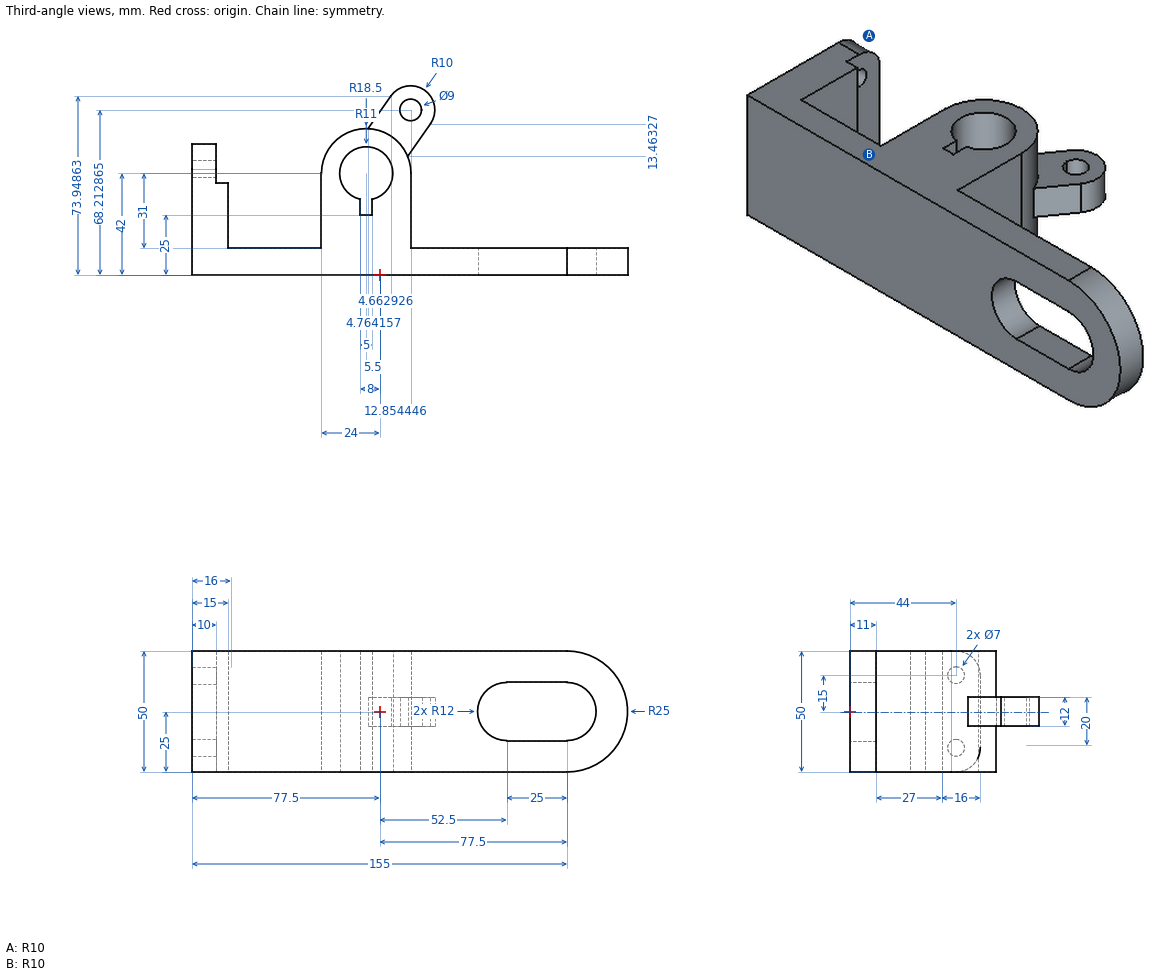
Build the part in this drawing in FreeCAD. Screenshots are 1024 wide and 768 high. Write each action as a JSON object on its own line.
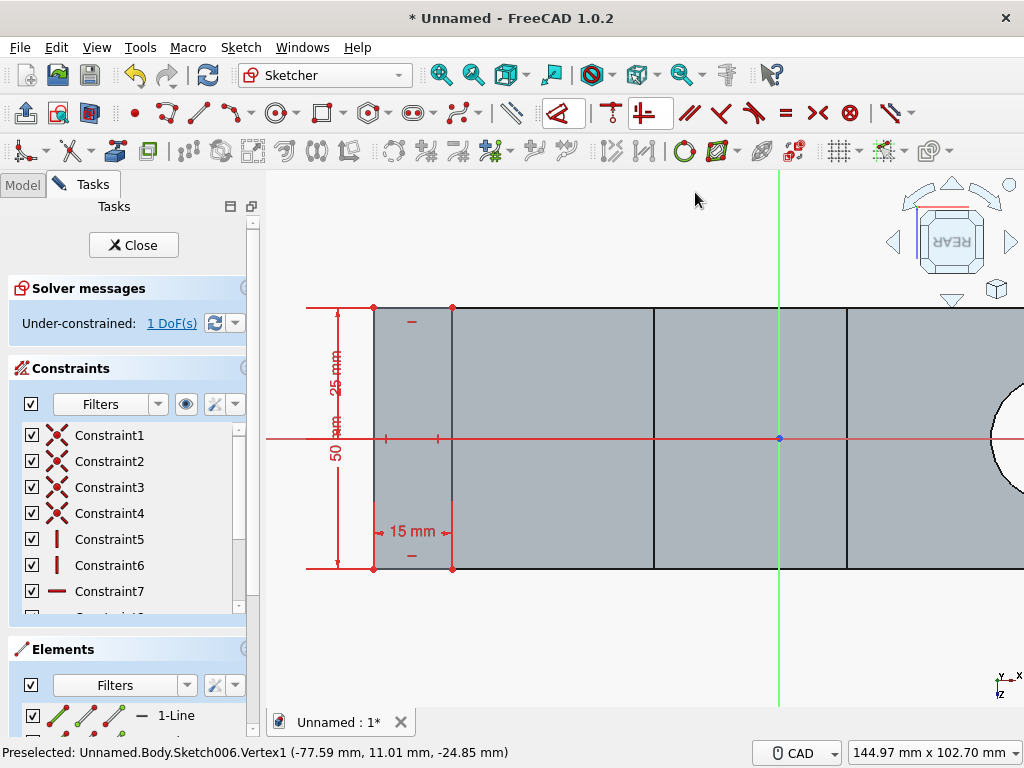
{"action": "left_click", "coordinate": [374, 308]}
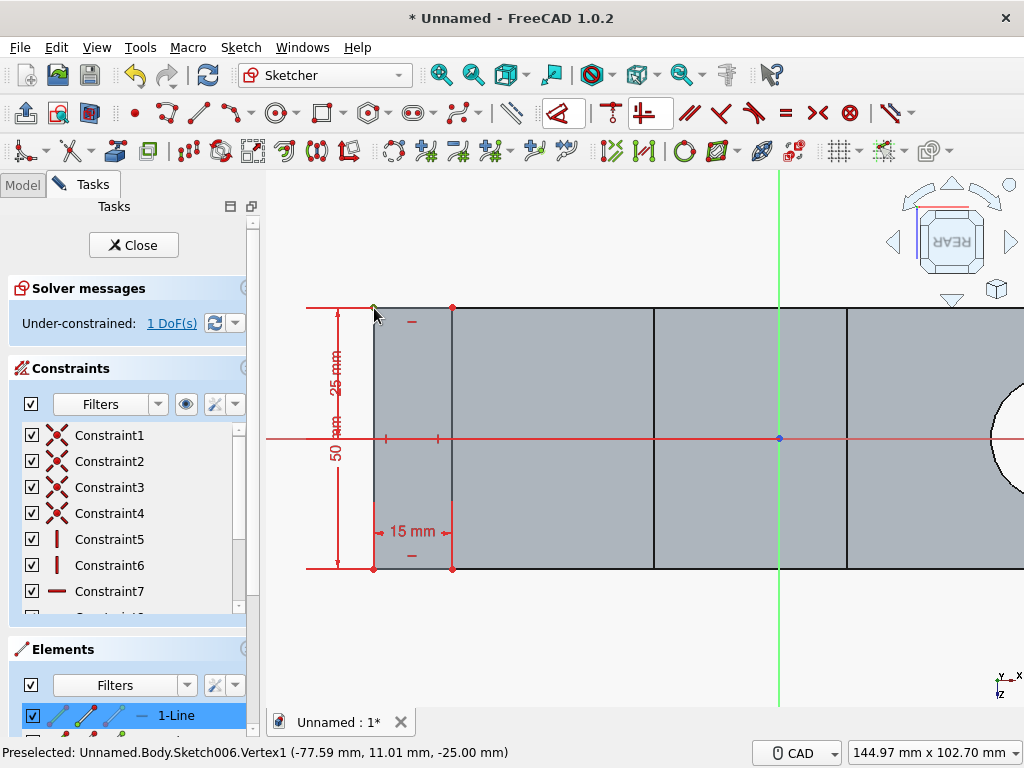
{"action": "left_click", "coordinate": [580, 114]}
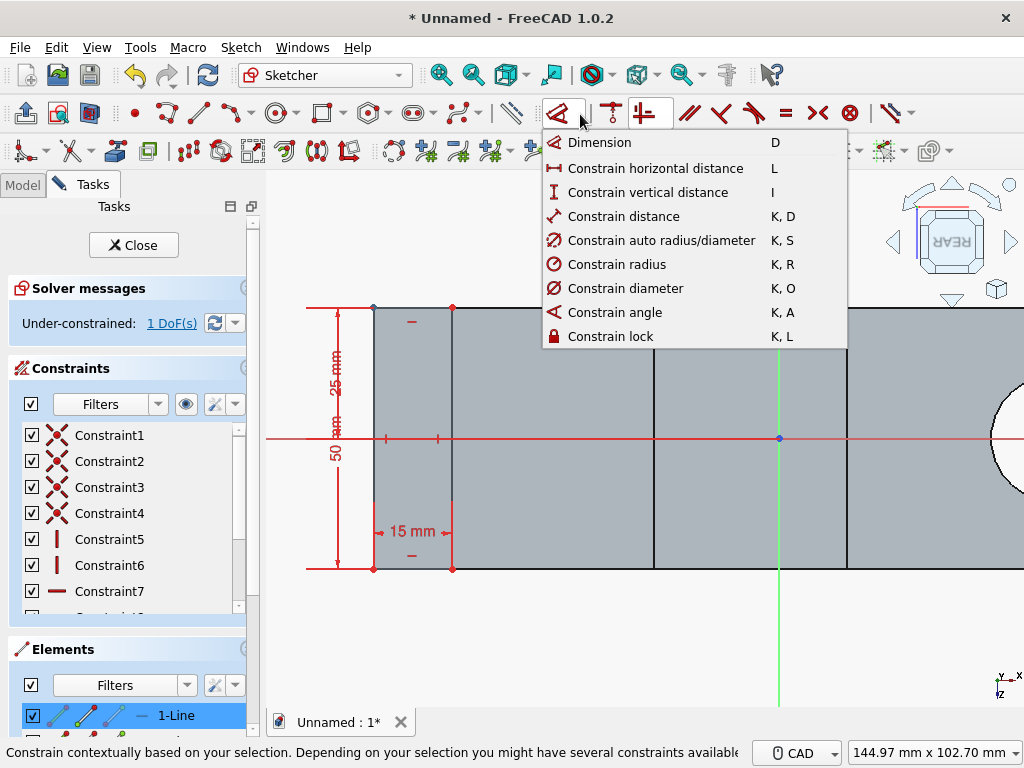
{"action": "left_click", "coordinate": [695, 168]}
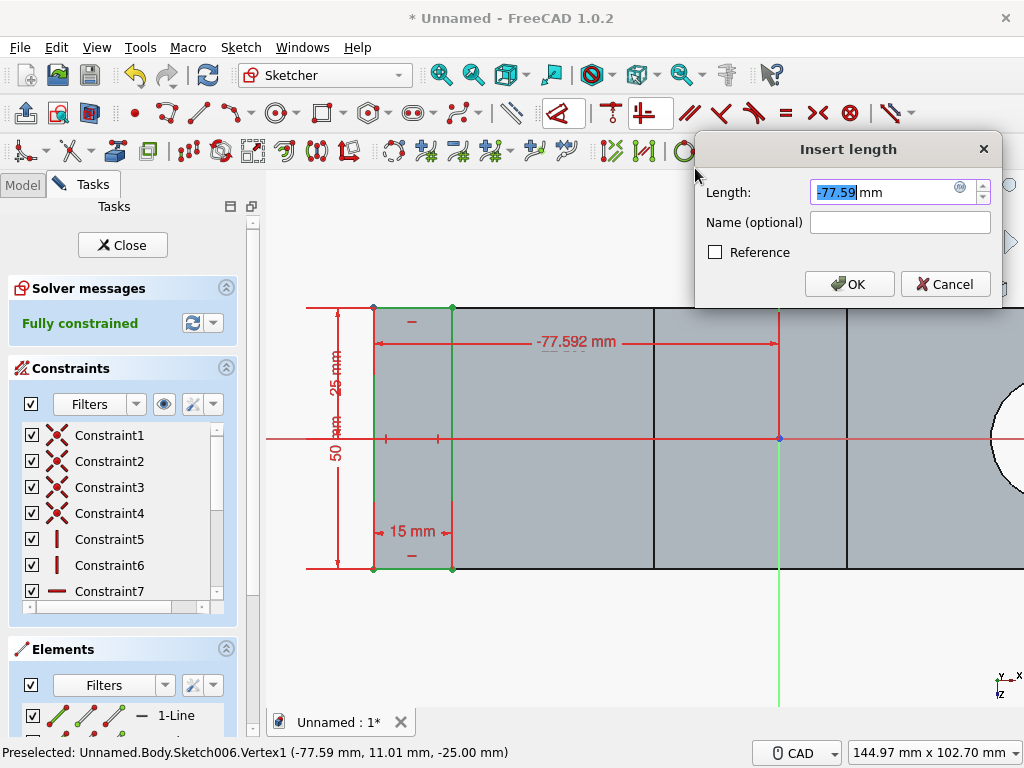
{"action": "type", "text": "-77.5"}
{"action": "key", "text": "Return"}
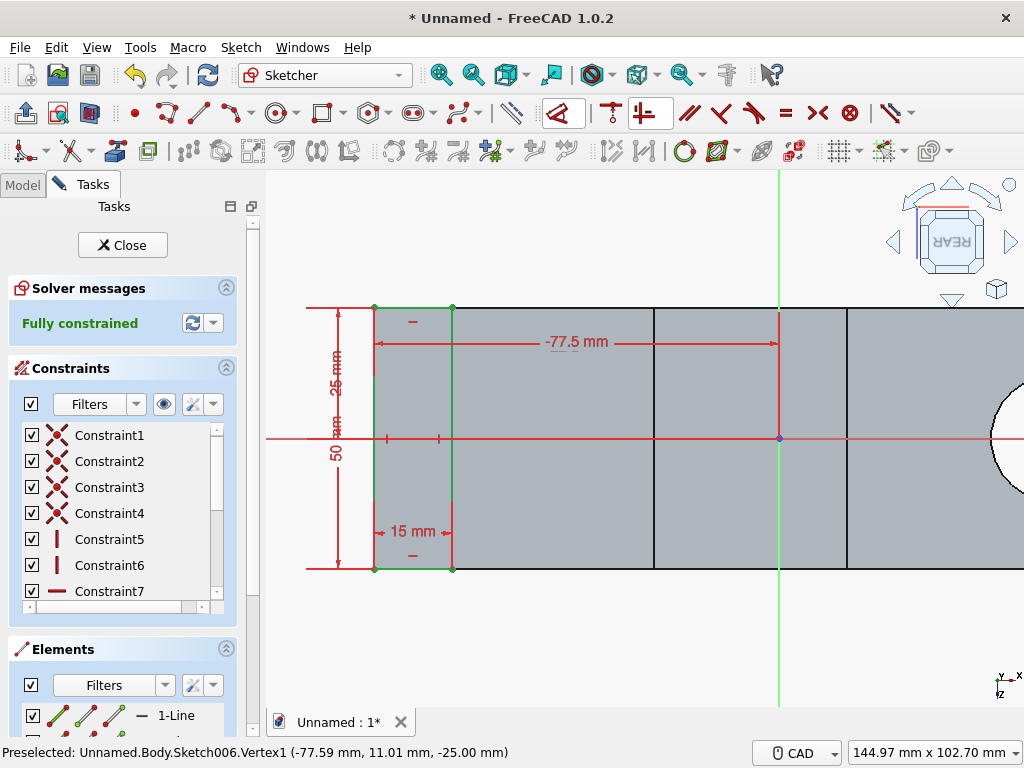
{"action": "left_click", "coordinate": [123, 245]}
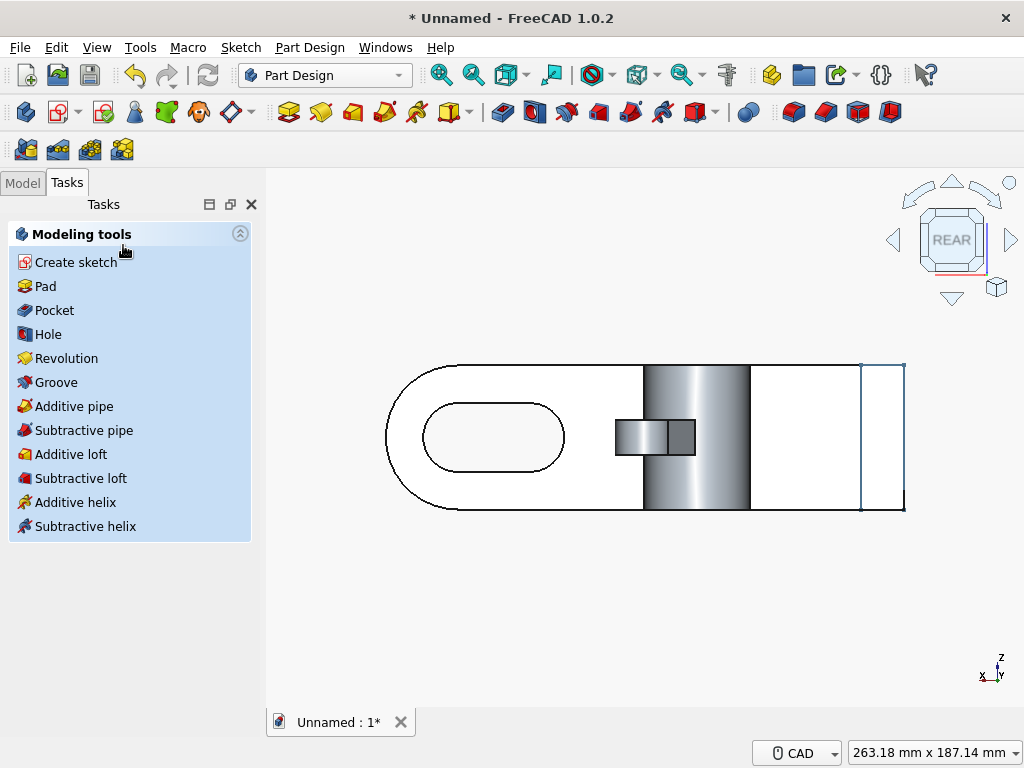
{"action": "left_click", "coordinate": [290, 112]}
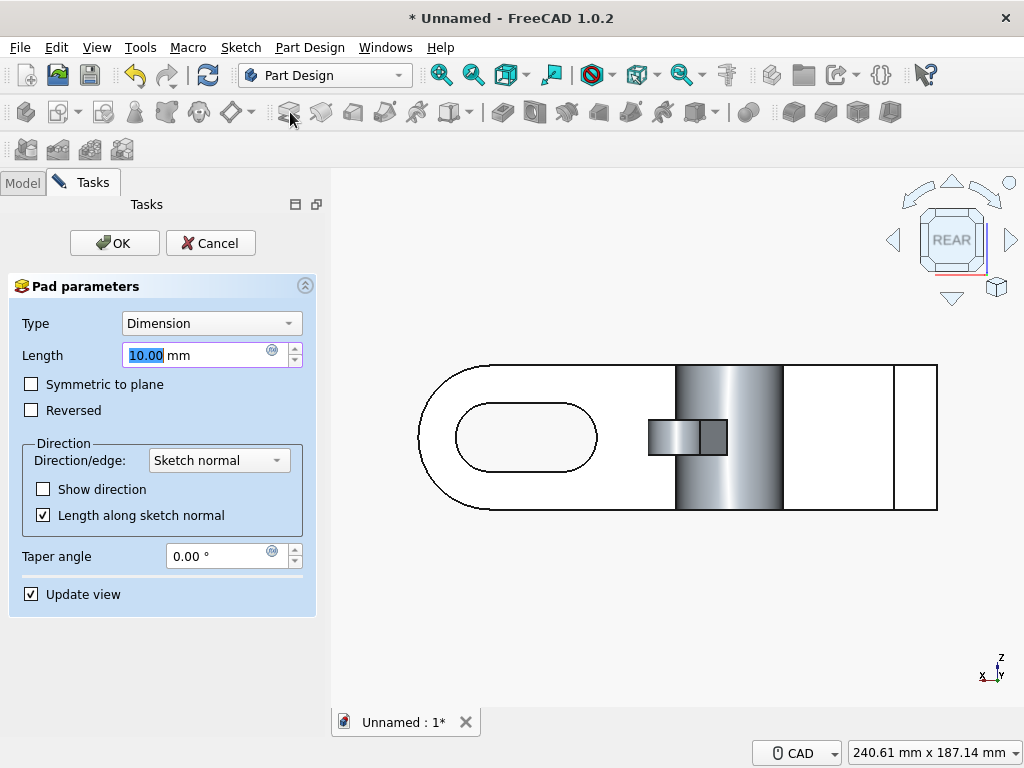
{"action": "type", "text": "27"}
{"action": "key", "text": "Tab"}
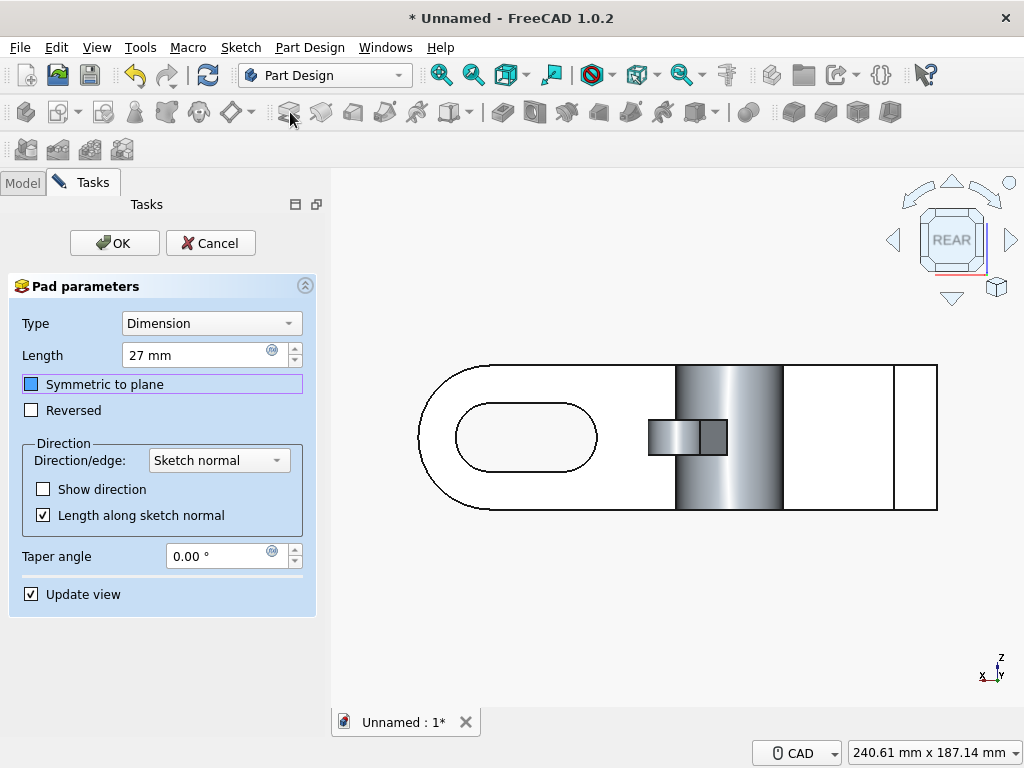
{"action": "left_click", "coordinate": [115, 243]}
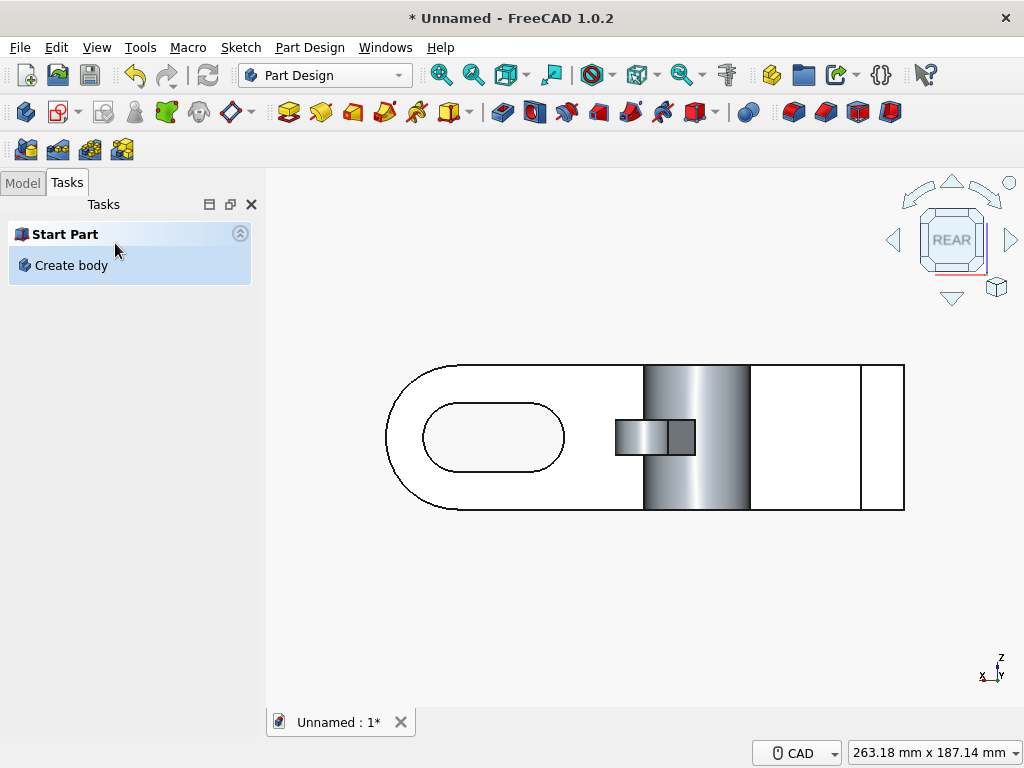
{"action": "left_click", "coordinate": [883, 395]}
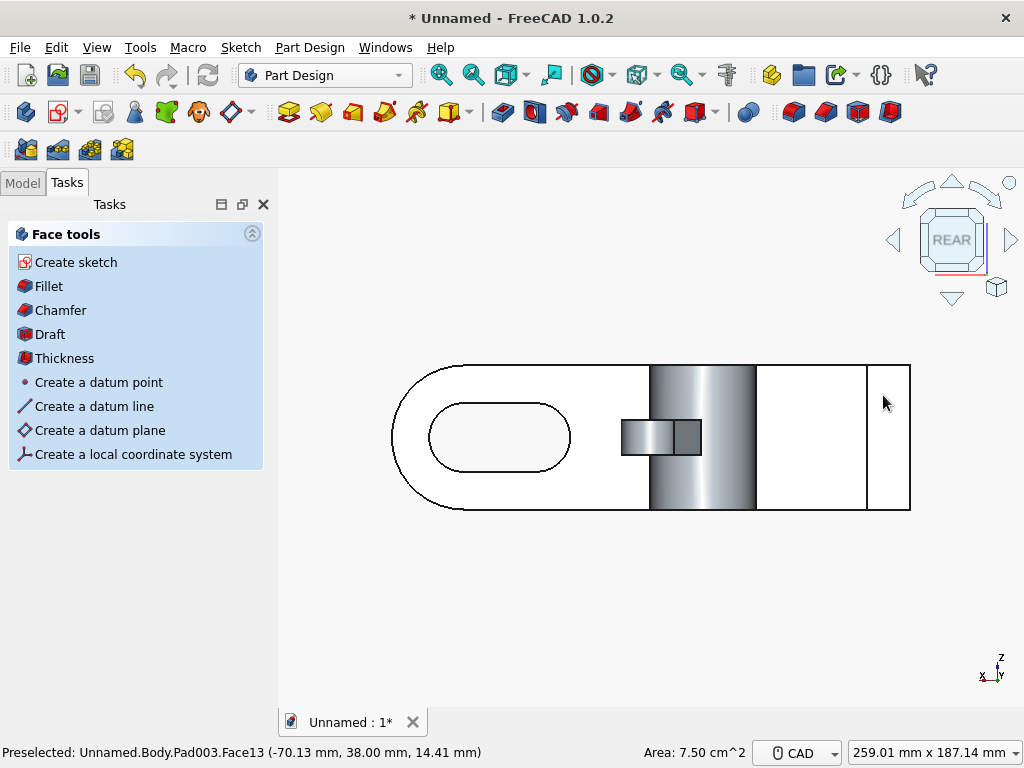
{"action": "left_click", "coordinate": [58, 112]}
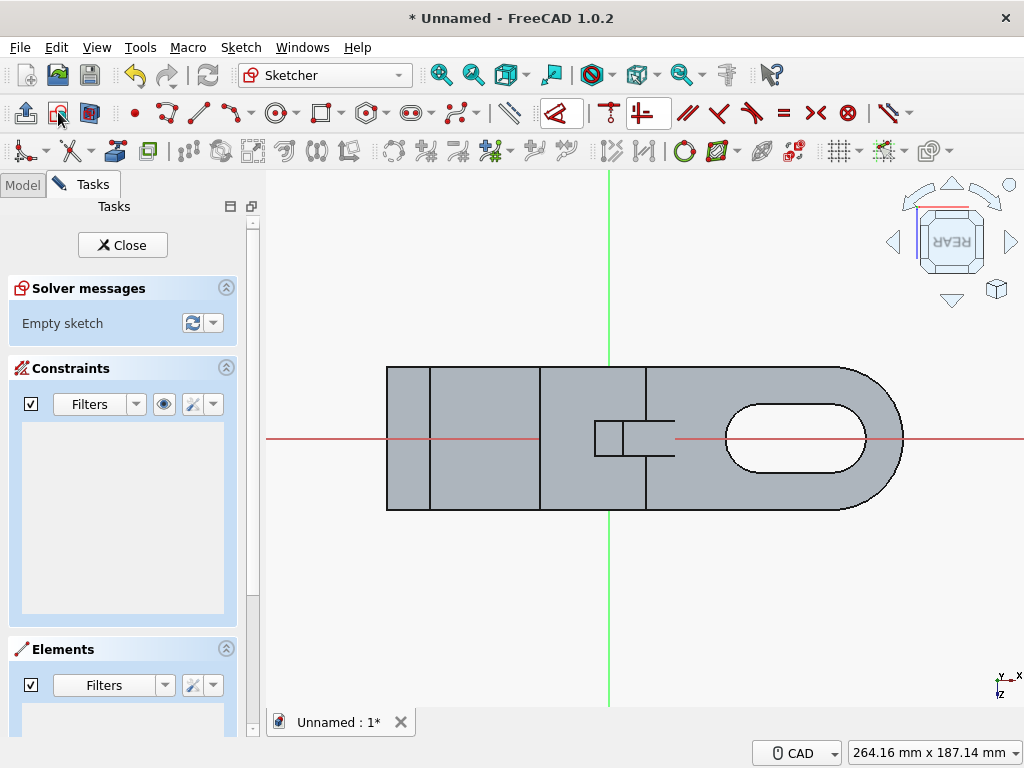
{"action": "scroll", "coordinate": [402, 438], "scroll_direction": "up", "scroll_amount": 3}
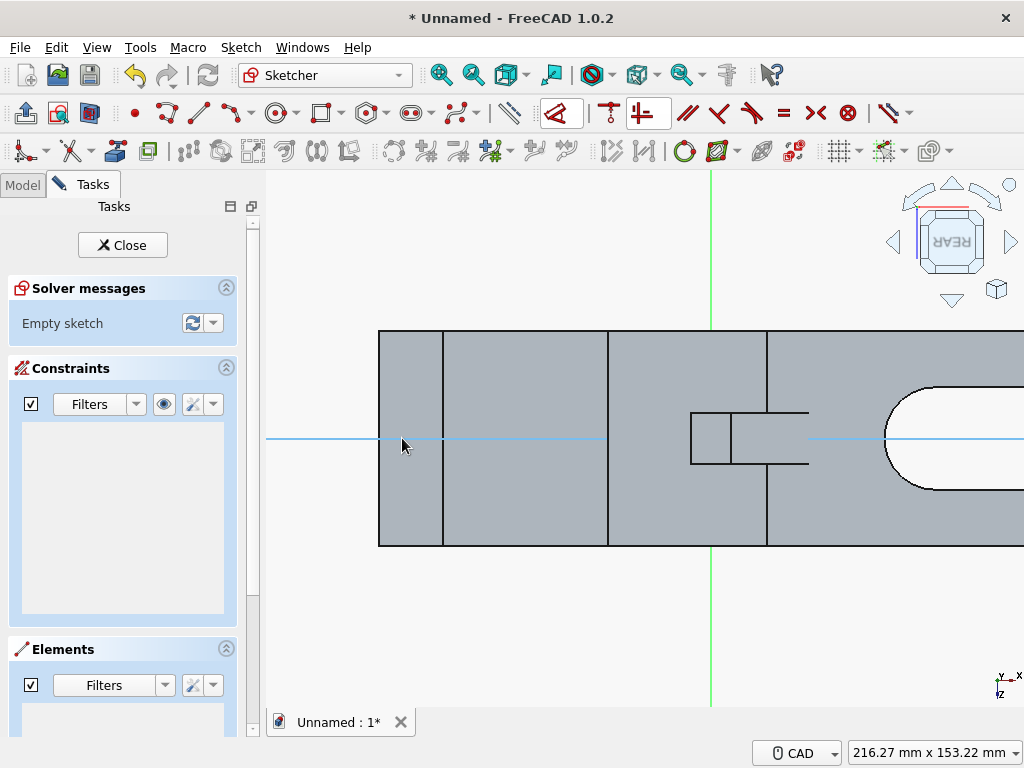
{"action": "left_click", "coordinate": [322, 114]}